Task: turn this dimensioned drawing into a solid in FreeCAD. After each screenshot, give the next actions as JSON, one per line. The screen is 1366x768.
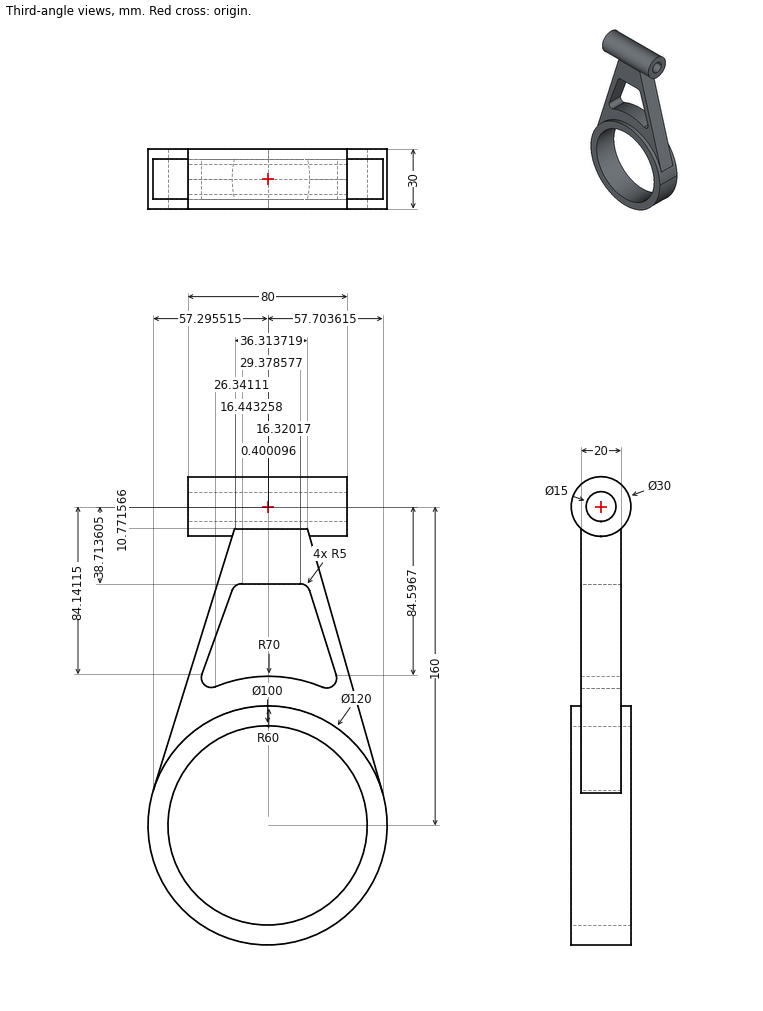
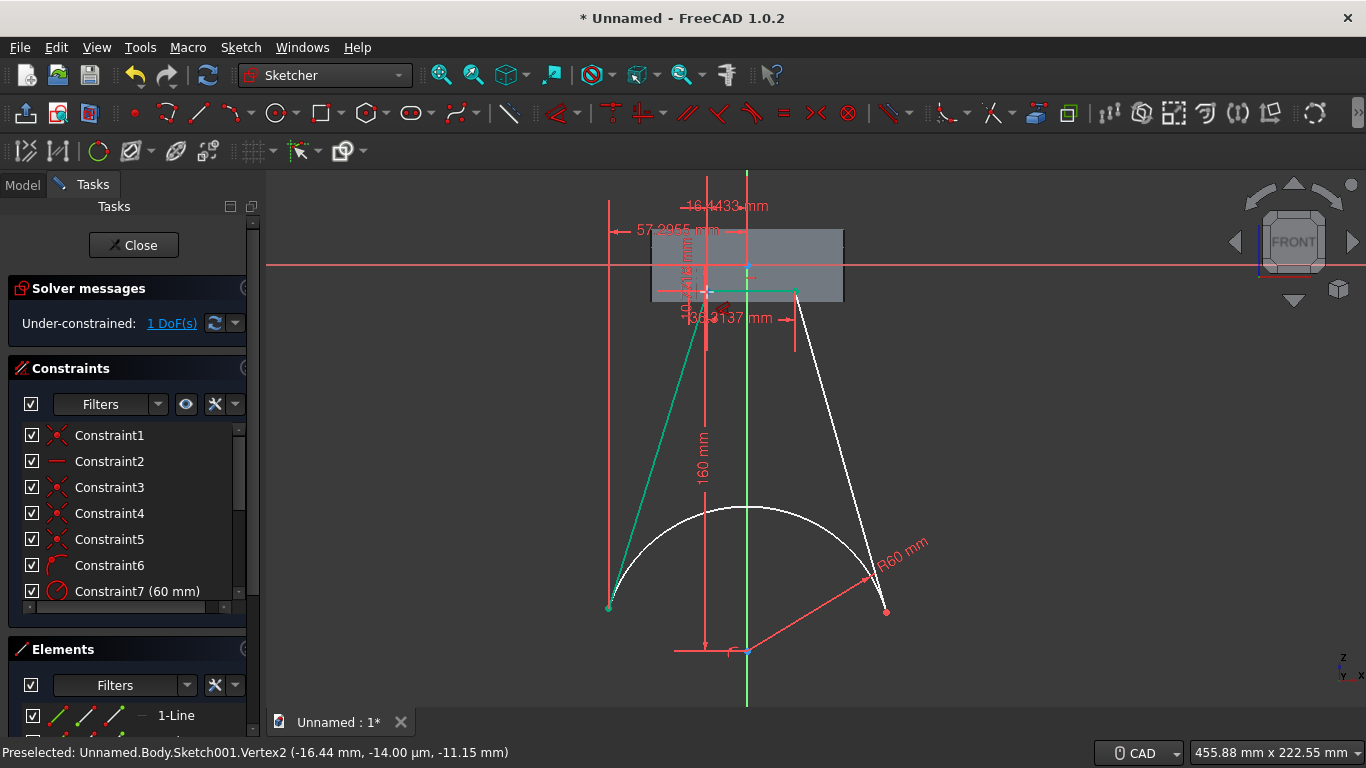
{"action": "left_click", "coordinate": [886, 612]}
{"action": "left_click", "coordinate": [817, 646]}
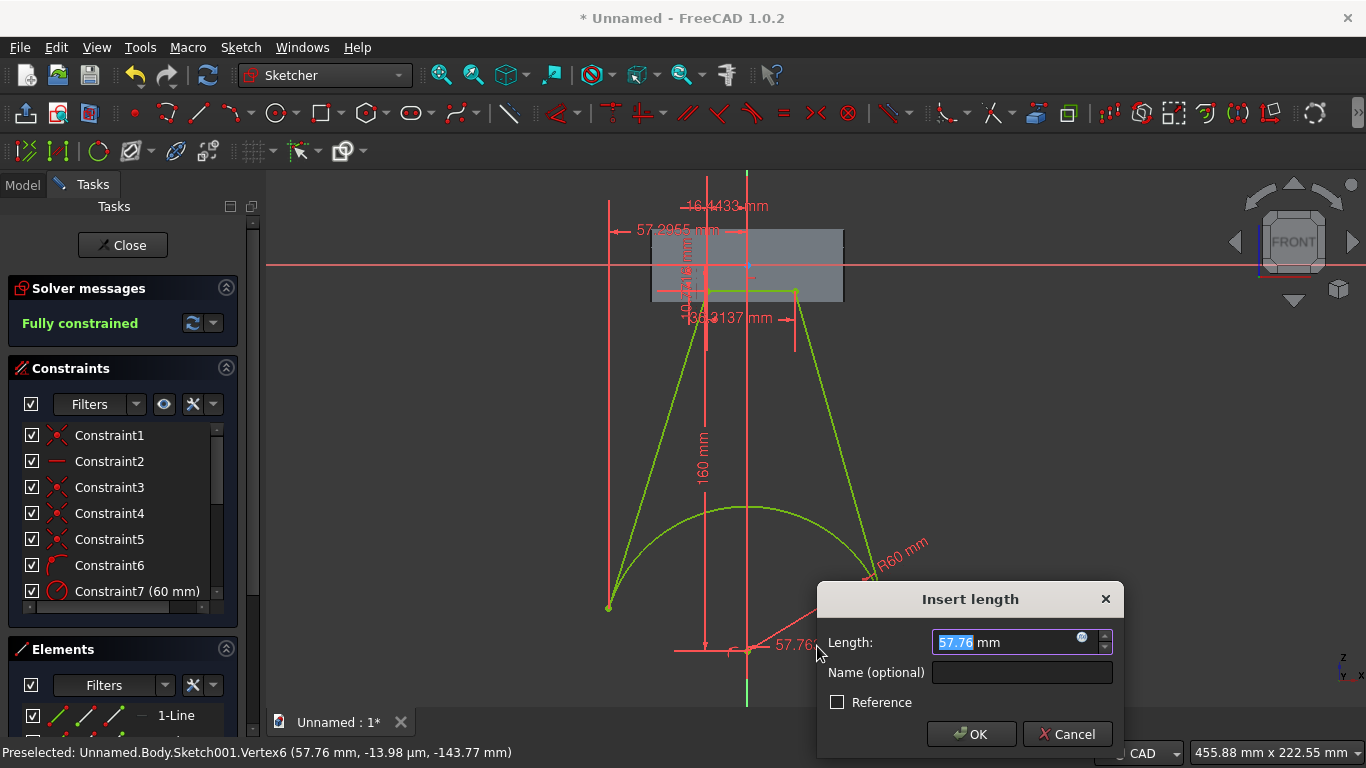
{"action": "type", "text": "57.703615"}
{"action": "key", "text": "Return"}
{"action": "key", "text": "Escape"}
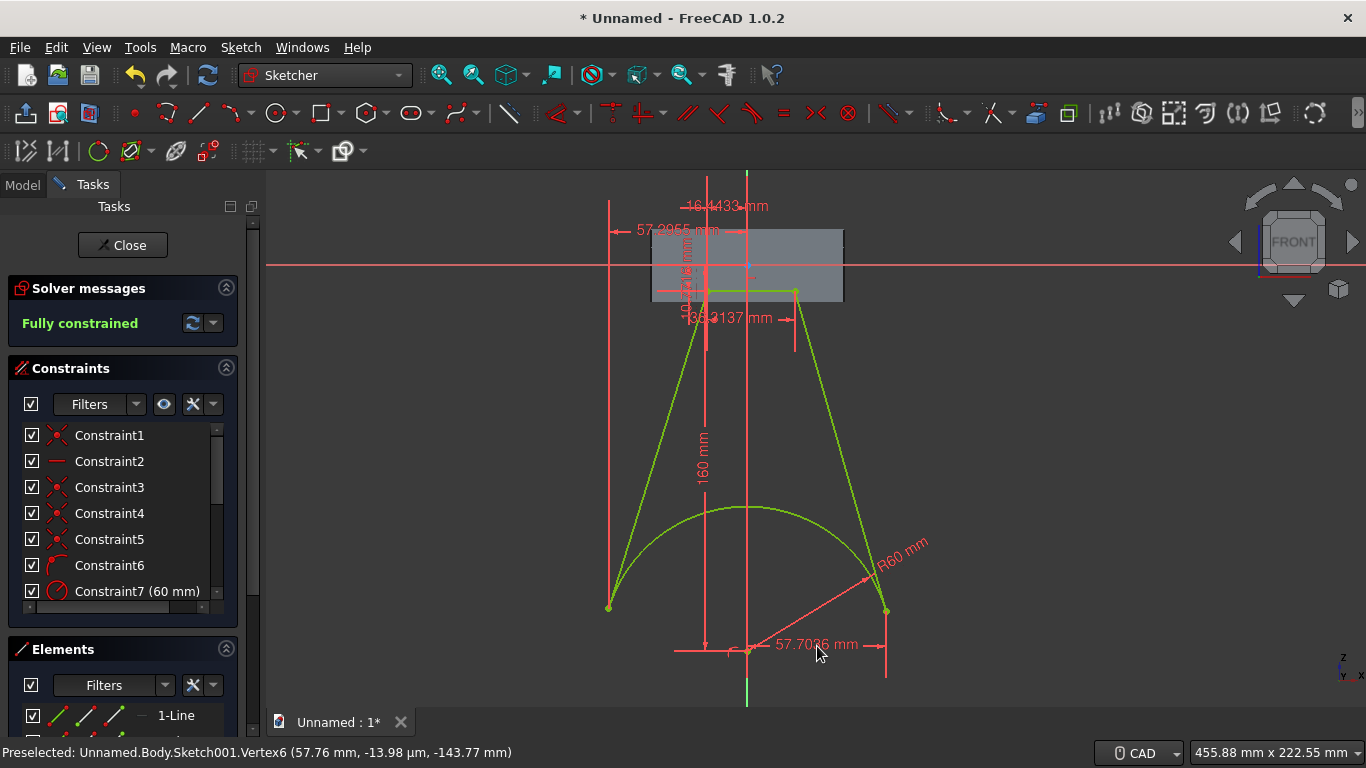
{"action": "left_click", "coordinate": [123, 245]}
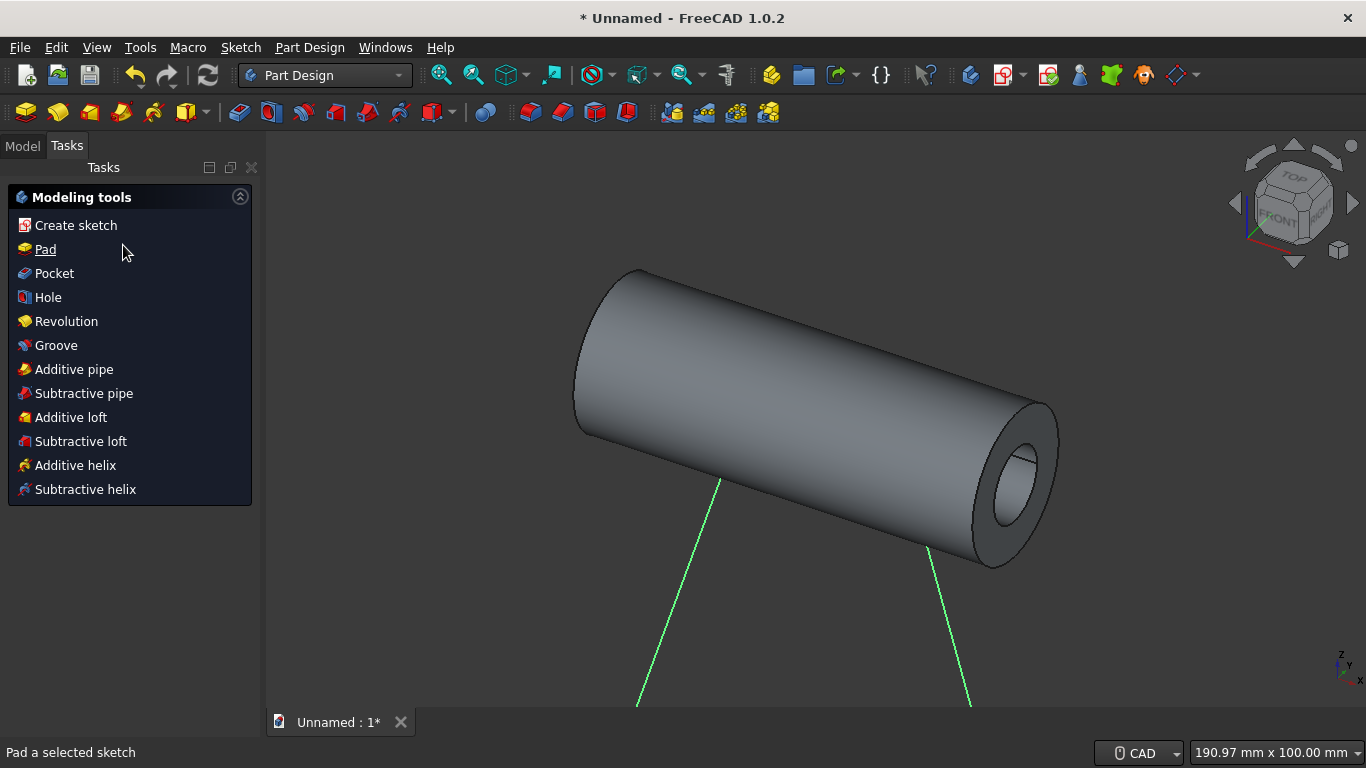
{"action": "left_click", "coordinate": [26, 112]}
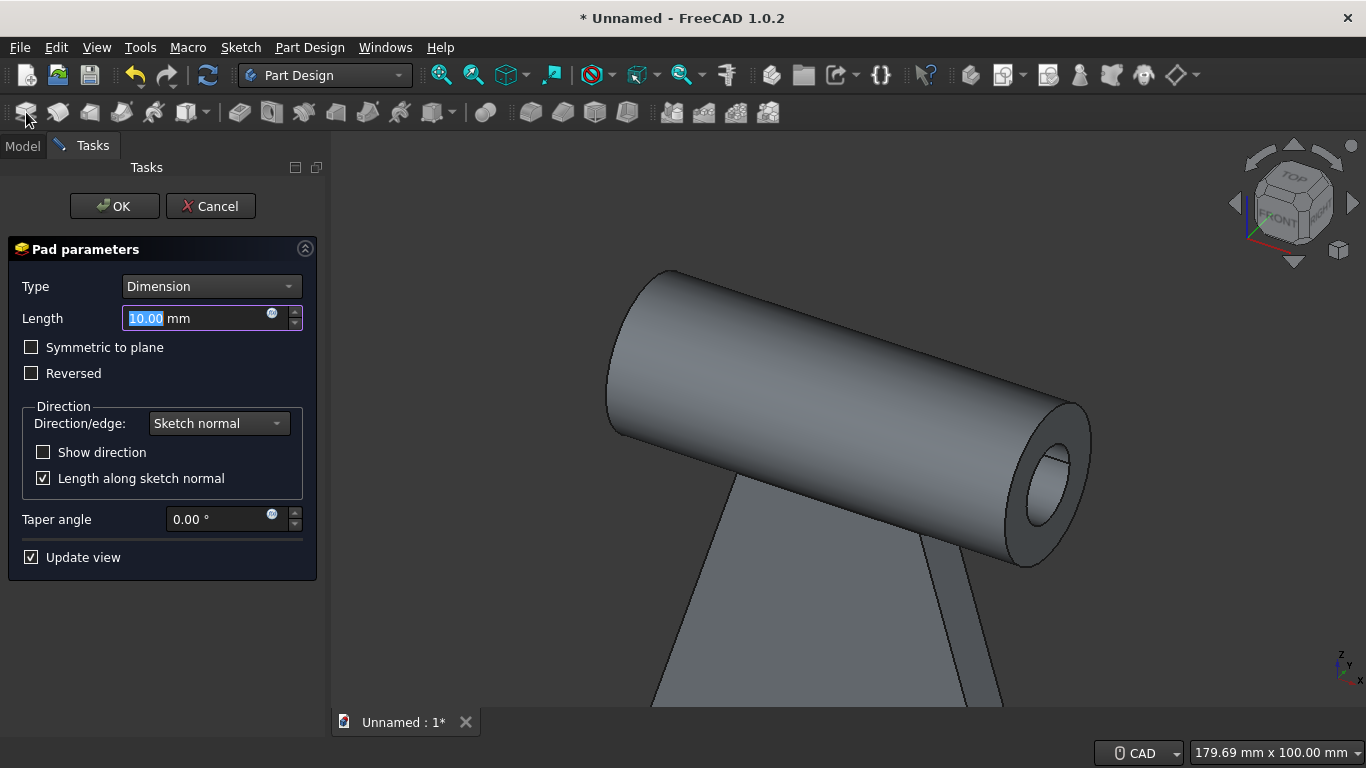
{"action": "type", "text": "20"}
{"action": "key", "text": "Tab"}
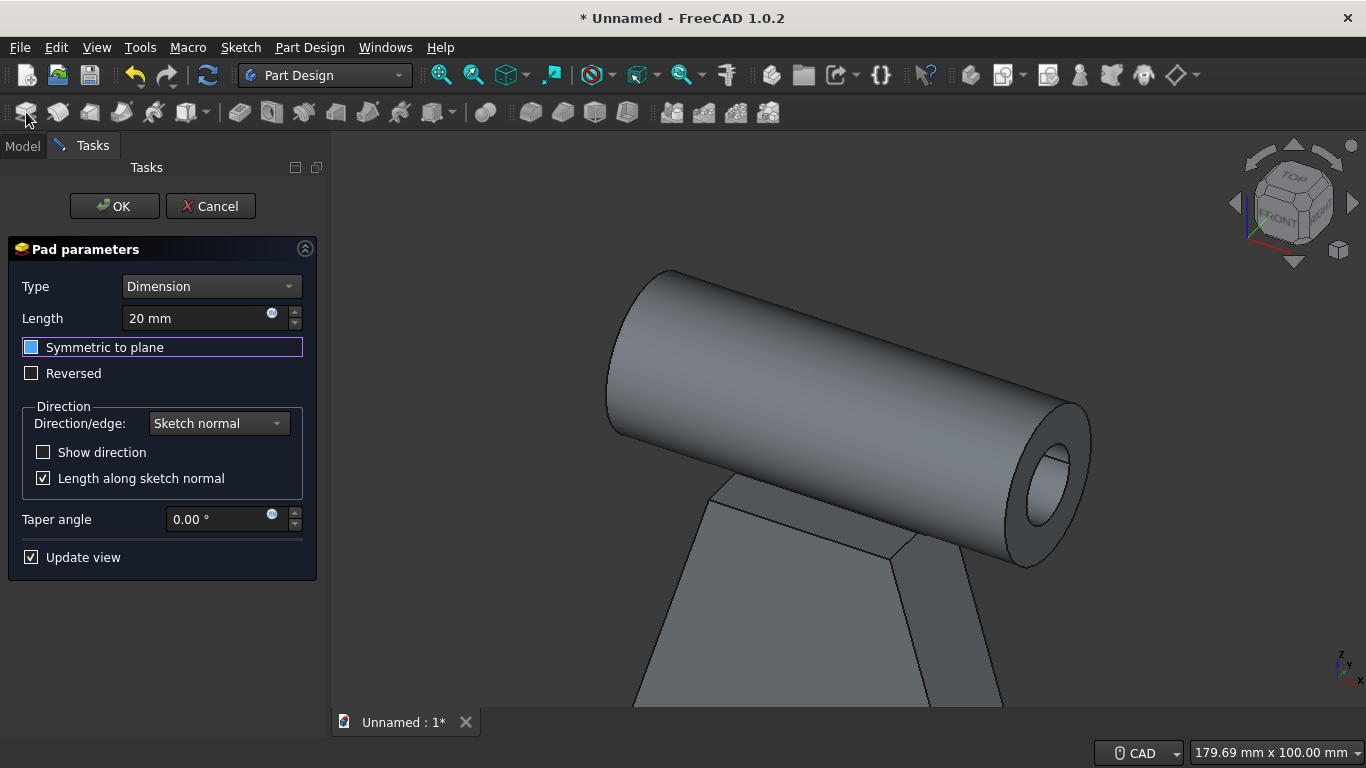
{"action": "left_click", "coordinate": [30, 347]}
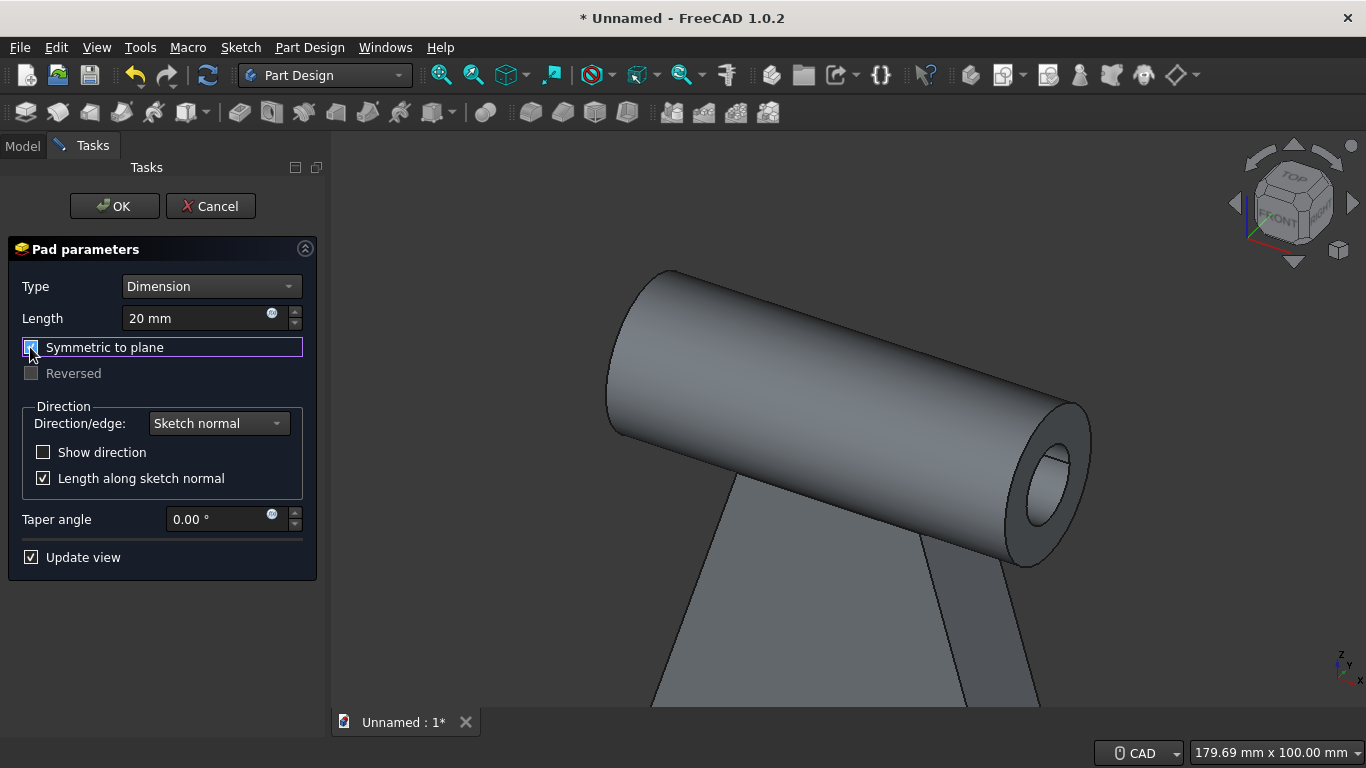
{"action": "left_click", "coordinate": [115, 206]}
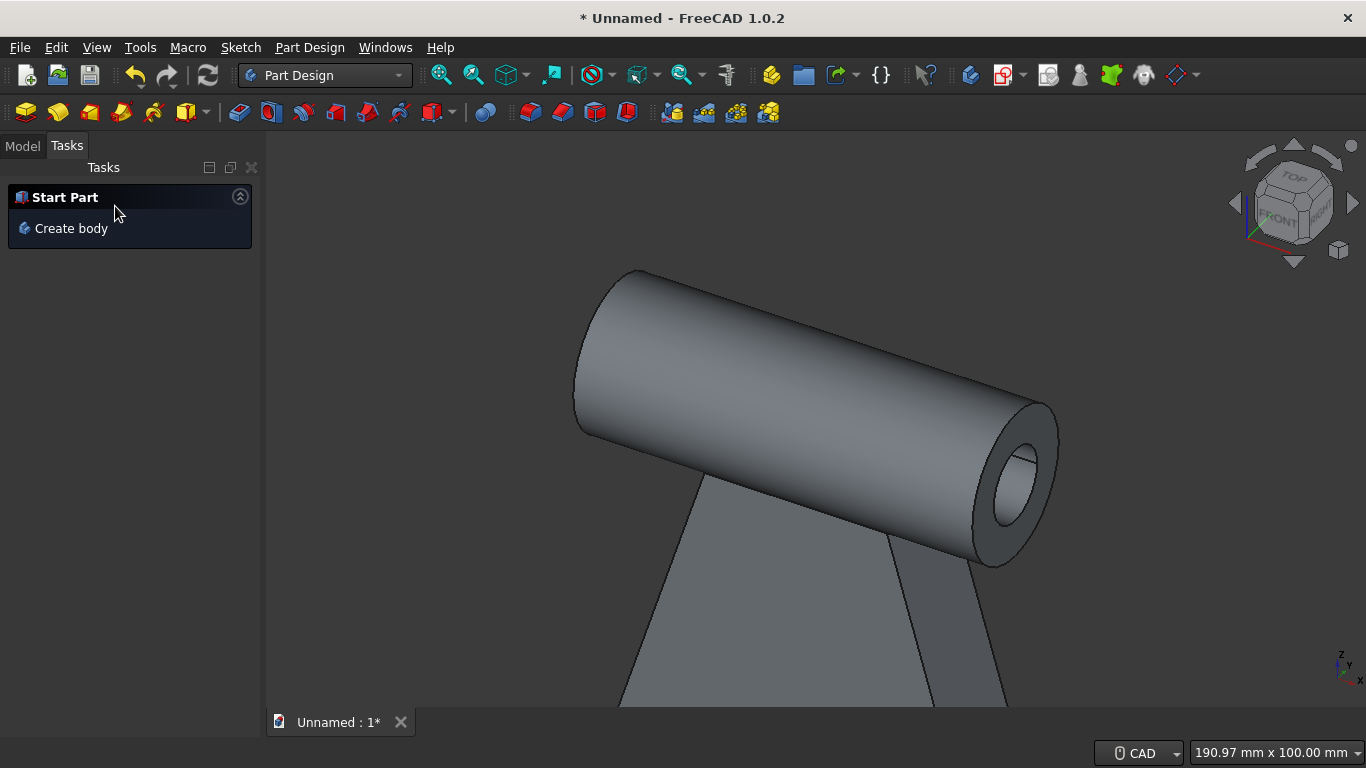
{"action": "left_click", "coordinate": [442, 76]}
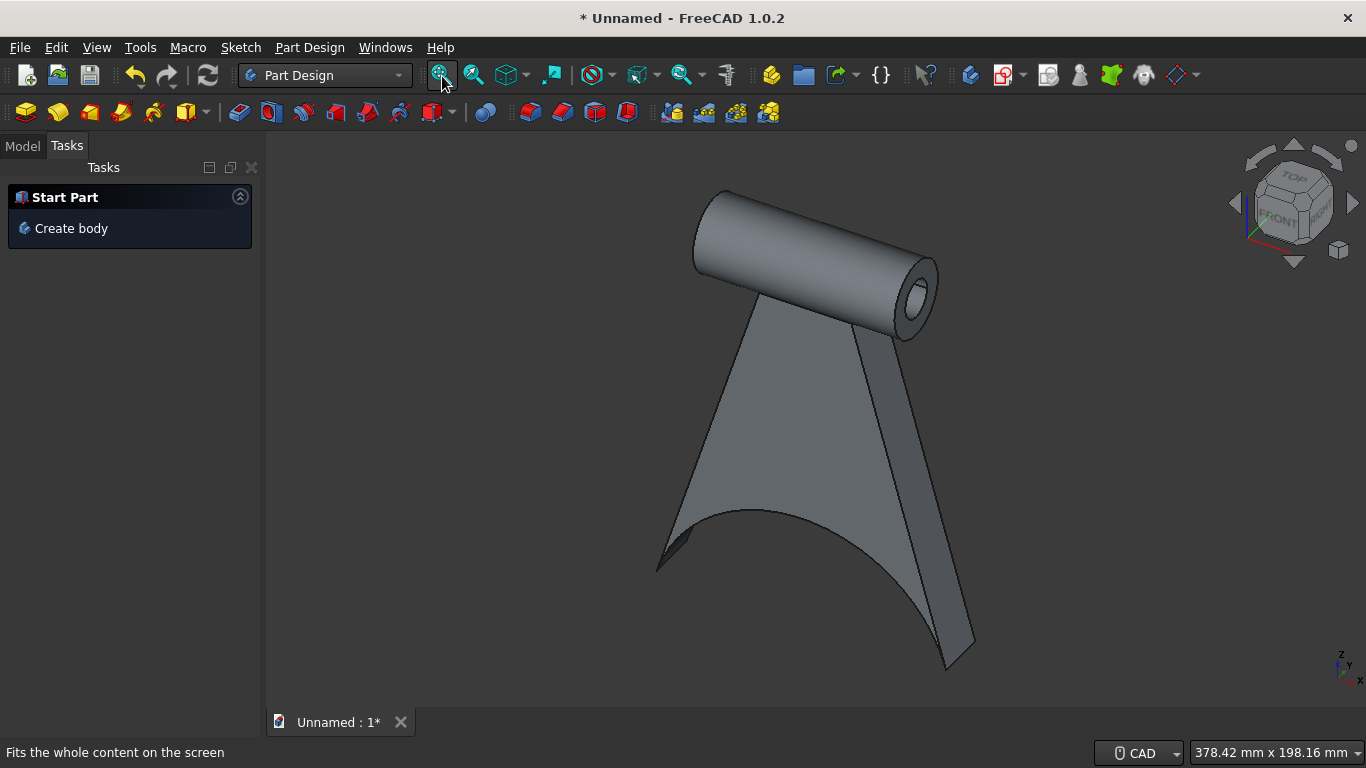
{"action": "left_click", "coordinate": [1004, 76]}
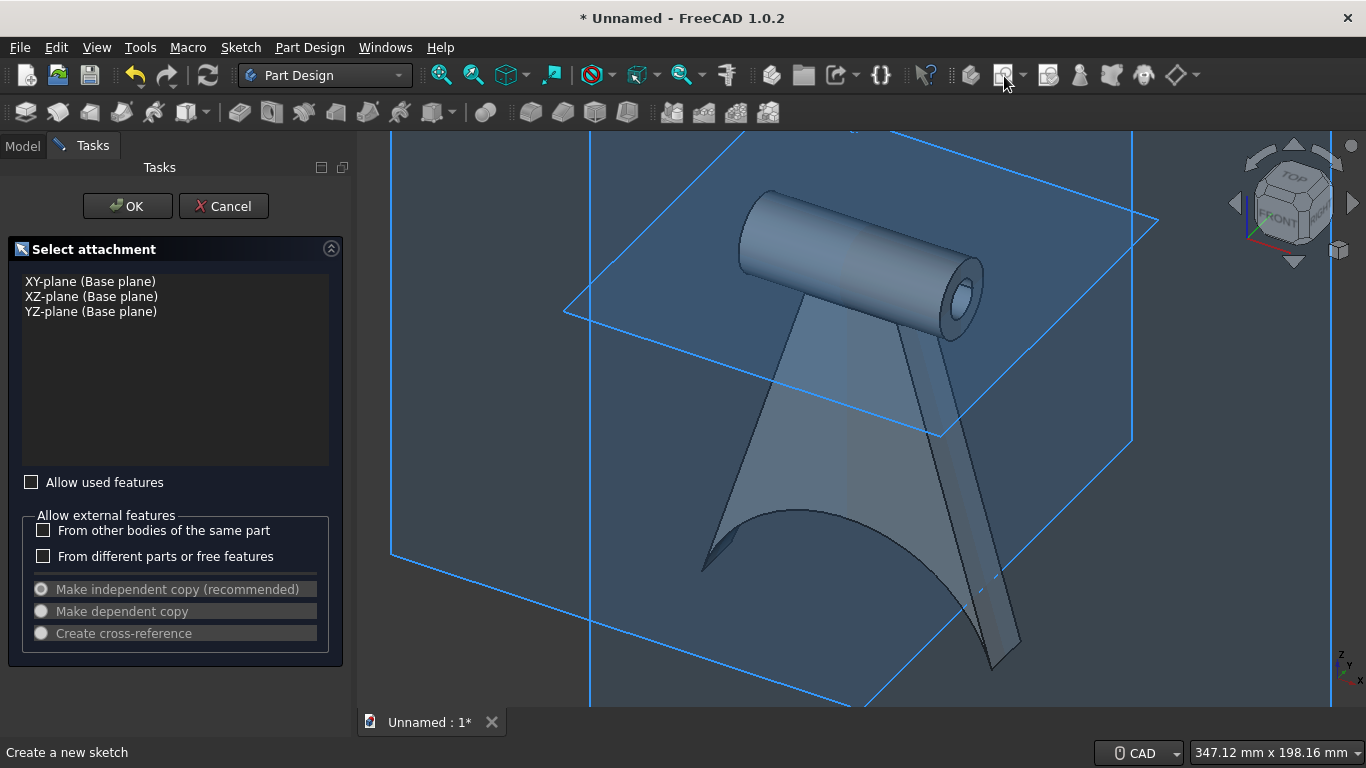
{"action": "left_click", "coordinate": [82, 296]}